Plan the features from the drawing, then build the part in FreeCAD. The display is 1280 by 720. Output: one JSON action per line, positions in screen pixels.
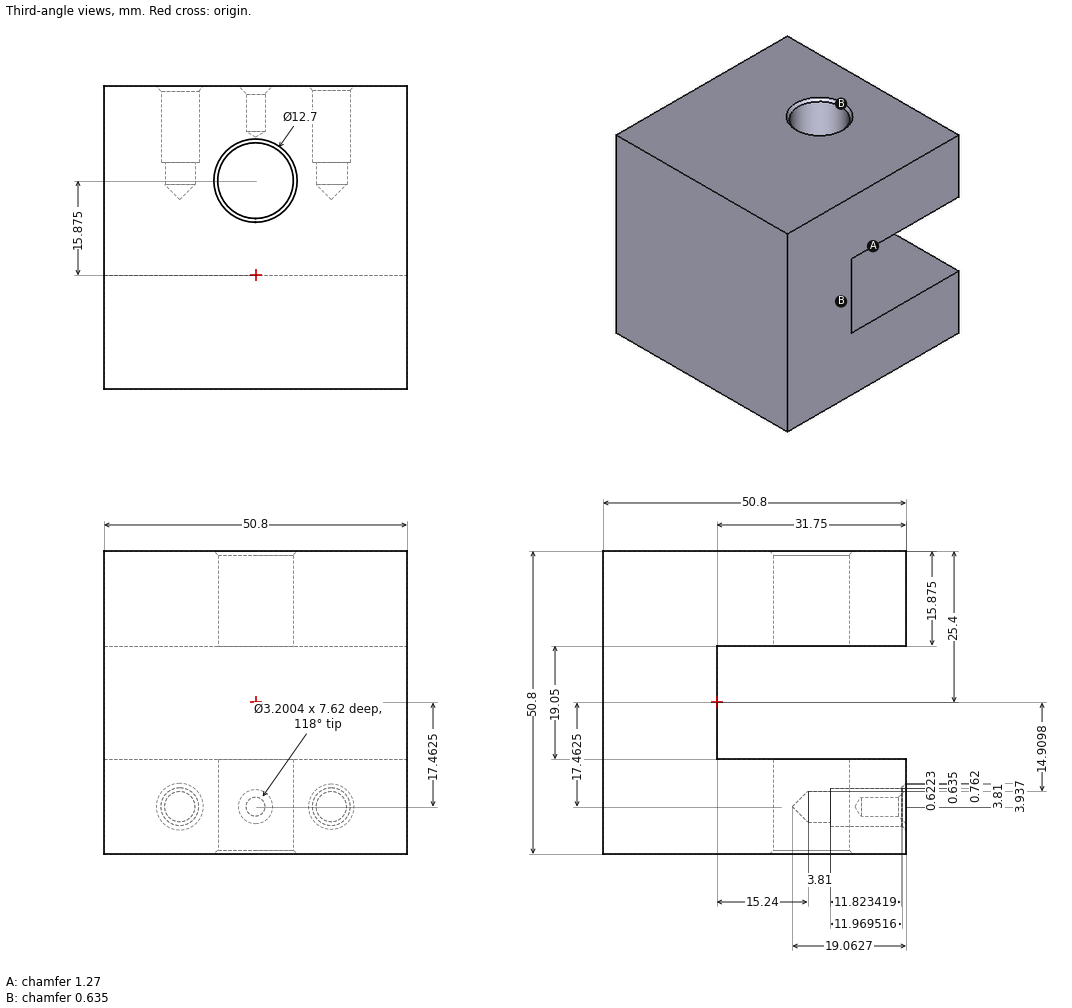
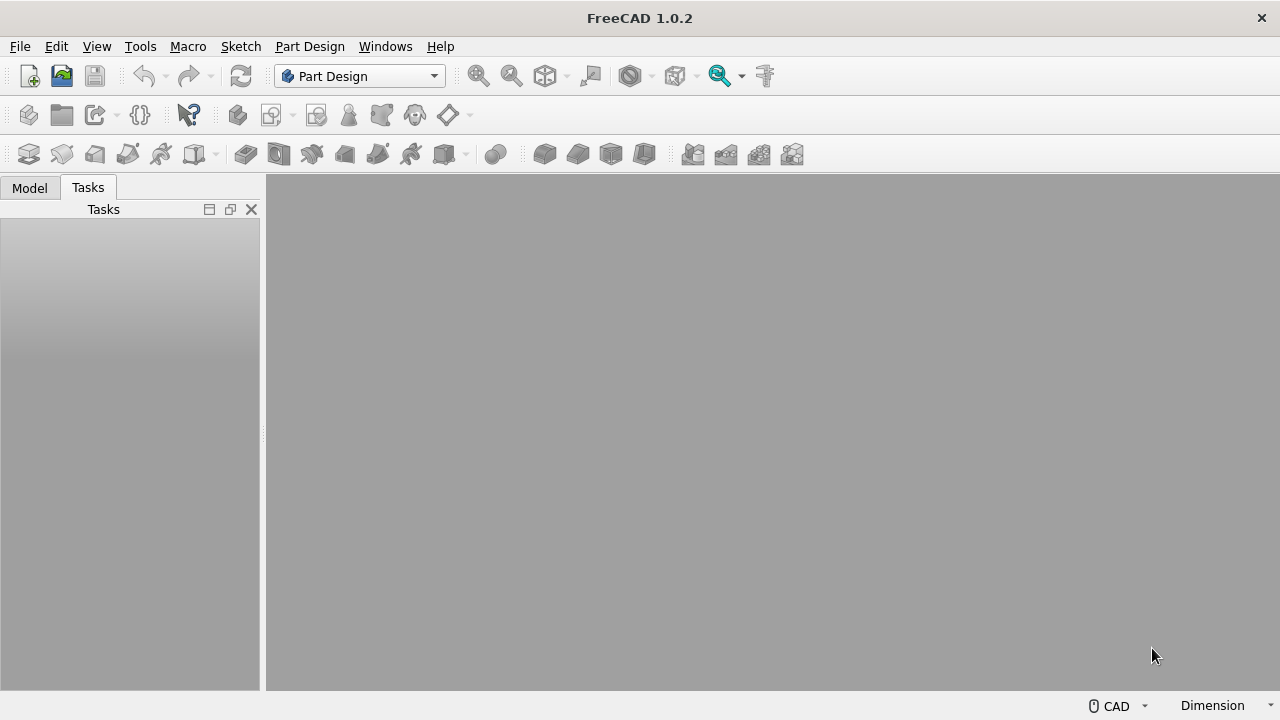
{"action": "left_click", "coordinate": [29, 76]}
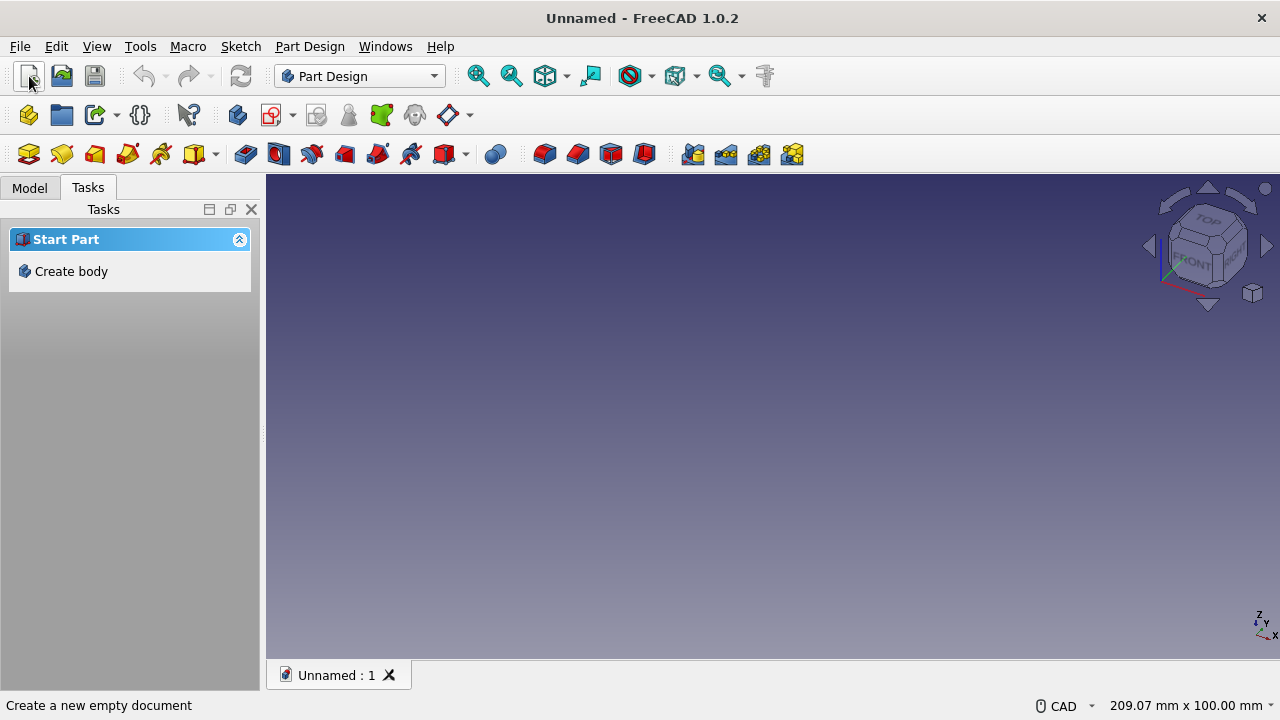
{"action": "left_click", "coordinate": [270, 116]}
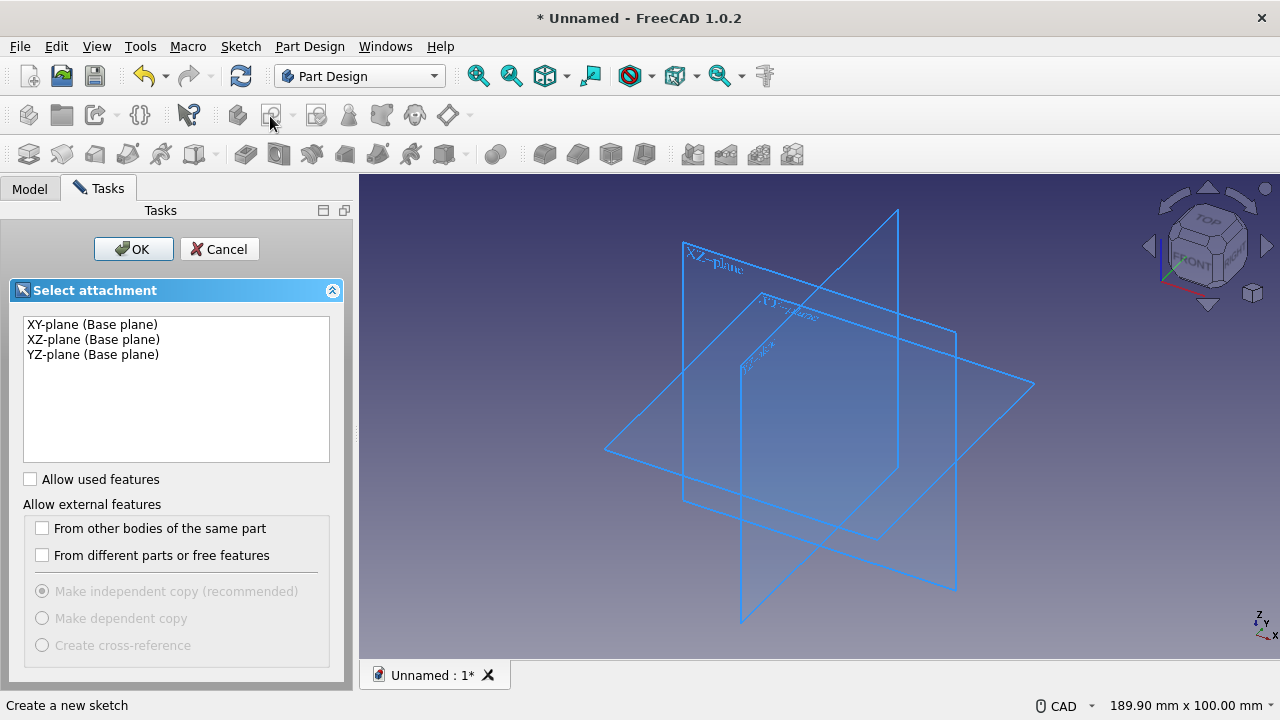
{"action": "left_click", "coordinate": [84, 354]}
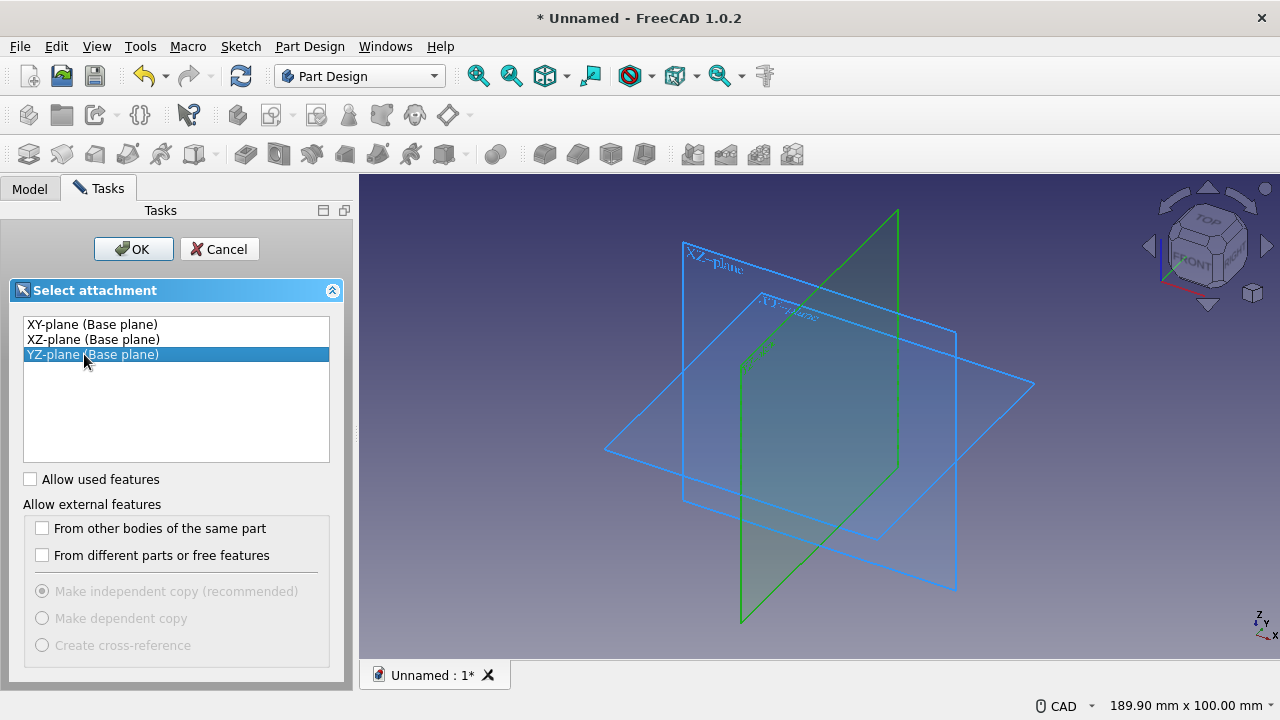
{"action": "left_click", "coordinate": [134, 249]}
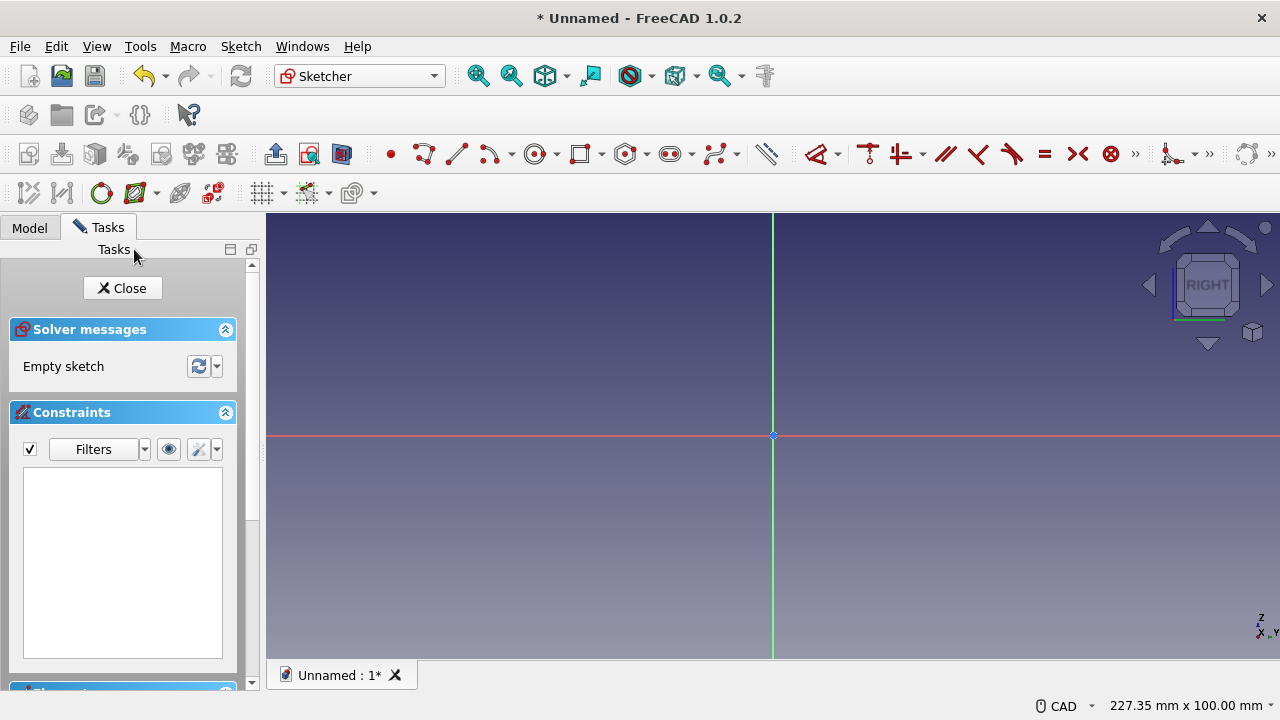
{"action": "left_click", "coordinate": [424, 154]}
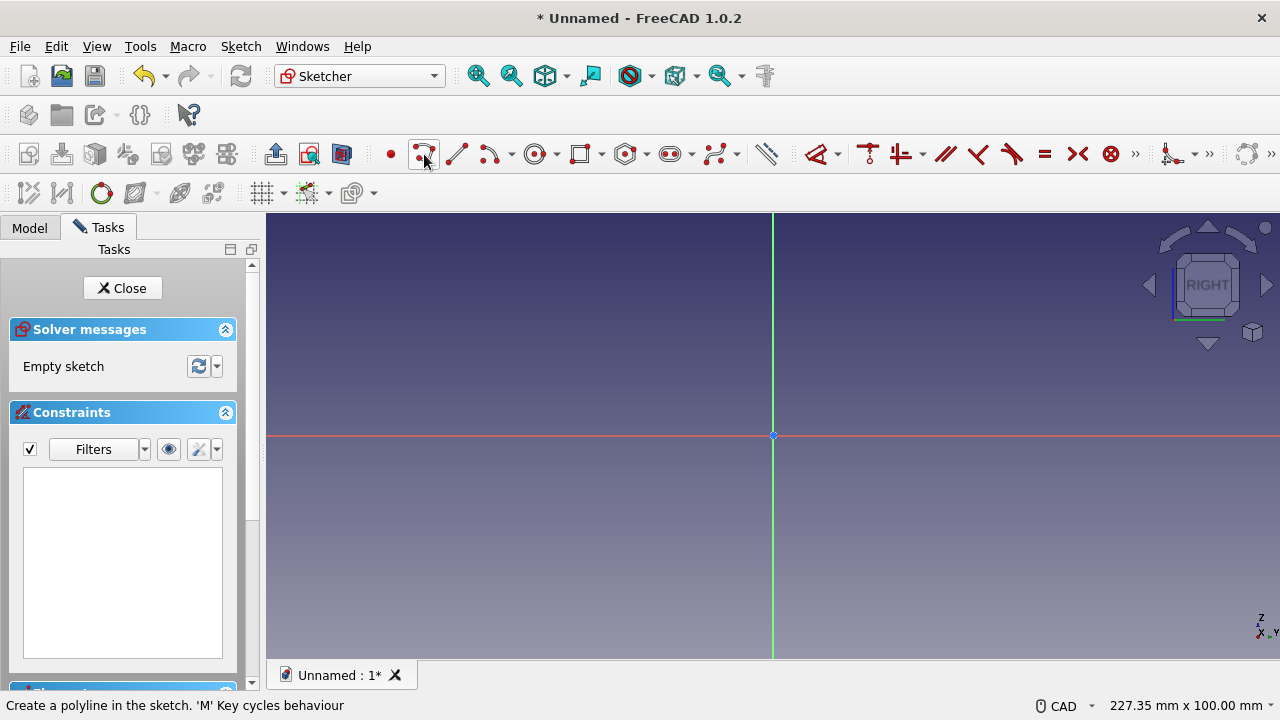
{"action": "left_click", "coordinate": [773, 478]}
{"action": "left_click", "coordinate": [782, 394]}
{"action": "left_click", "coordinate": [915, 394]}
{"action": "left_click", "coordinate": [915, 323]}
{"action": "left_click", "coordinate": [688, 323]}
{"action": "left_click", "coordinate": [688, 549]}
{"action": "left_click", "coordinate": [915, 549]}
{"action": "left_click", "coordinate": [915, 478]}
{"action": "left_click", "coordinate": [773, 479]}
{"action": "key", "text": "Escape"}
{"action": "key", "text": "Escape"}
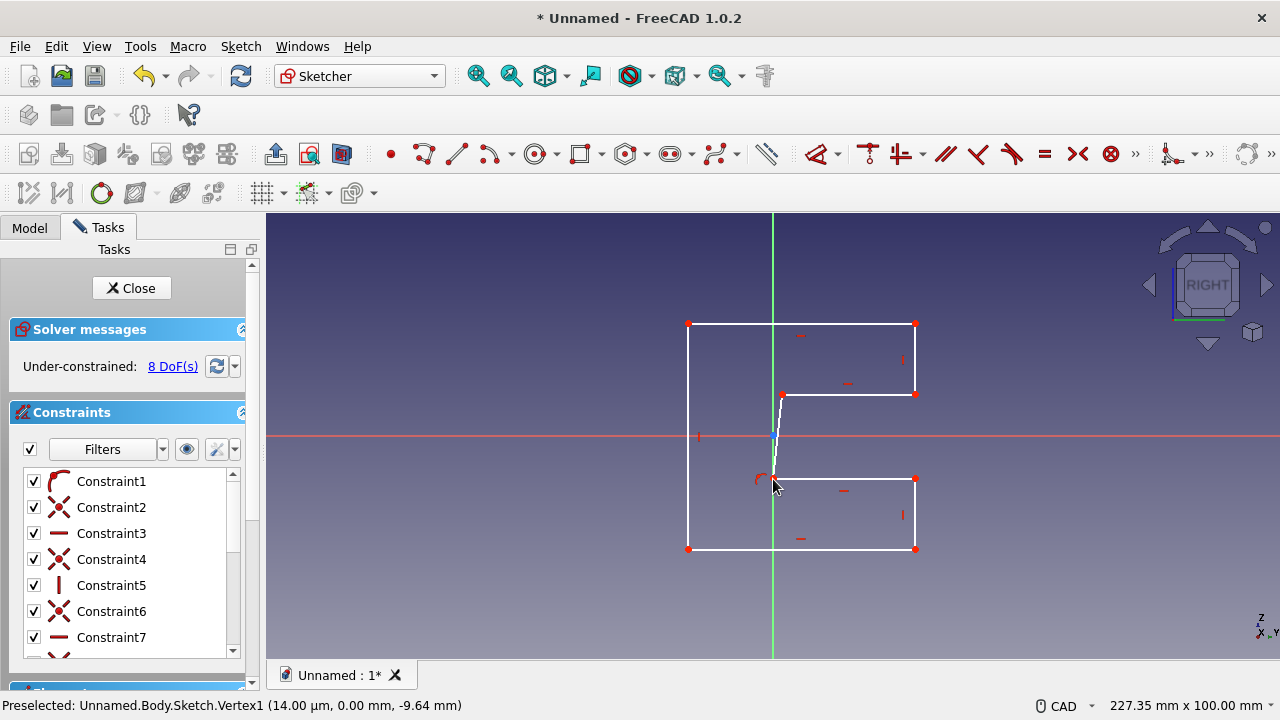
{"action": "left_click", "coordinate": [776, 454]}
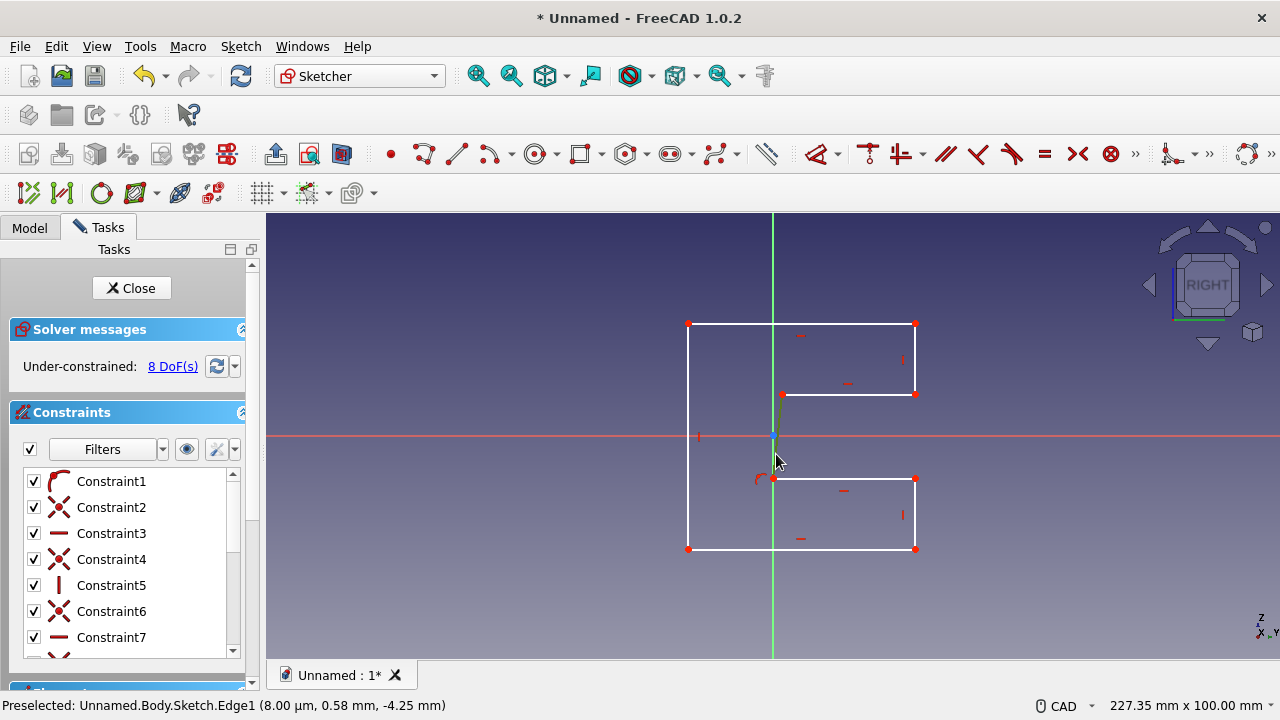
{"action": "key", "text": "v"}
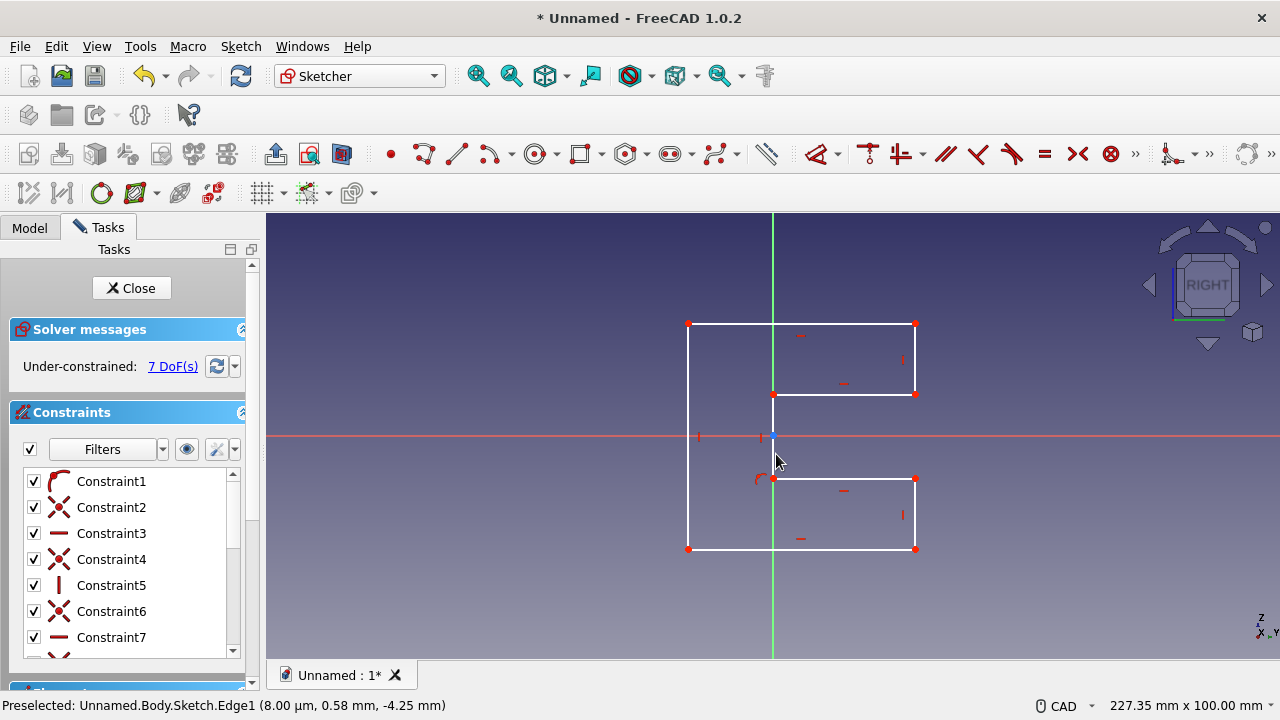
{"action": "left_click", "coordinate": [816, 154]}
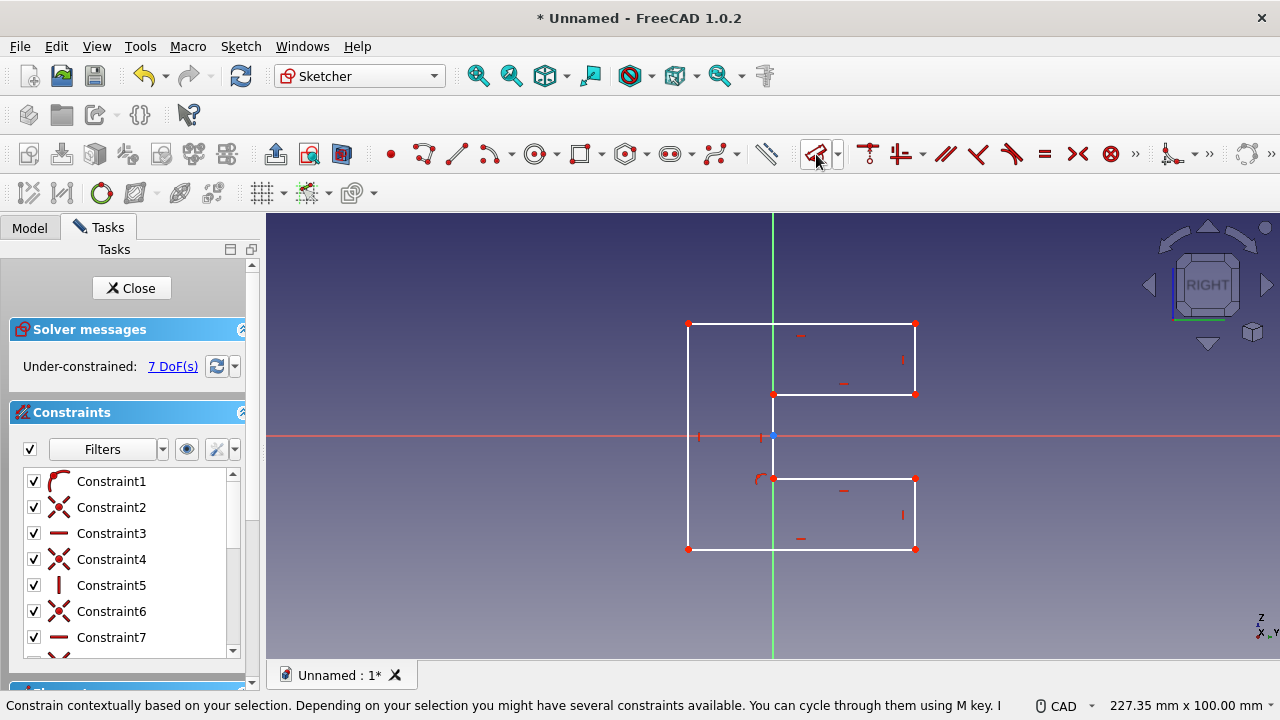
{"action": "left_click", "coordinate": [847, 324]}
{"action": "left_click", "coordinate": [802, 290]}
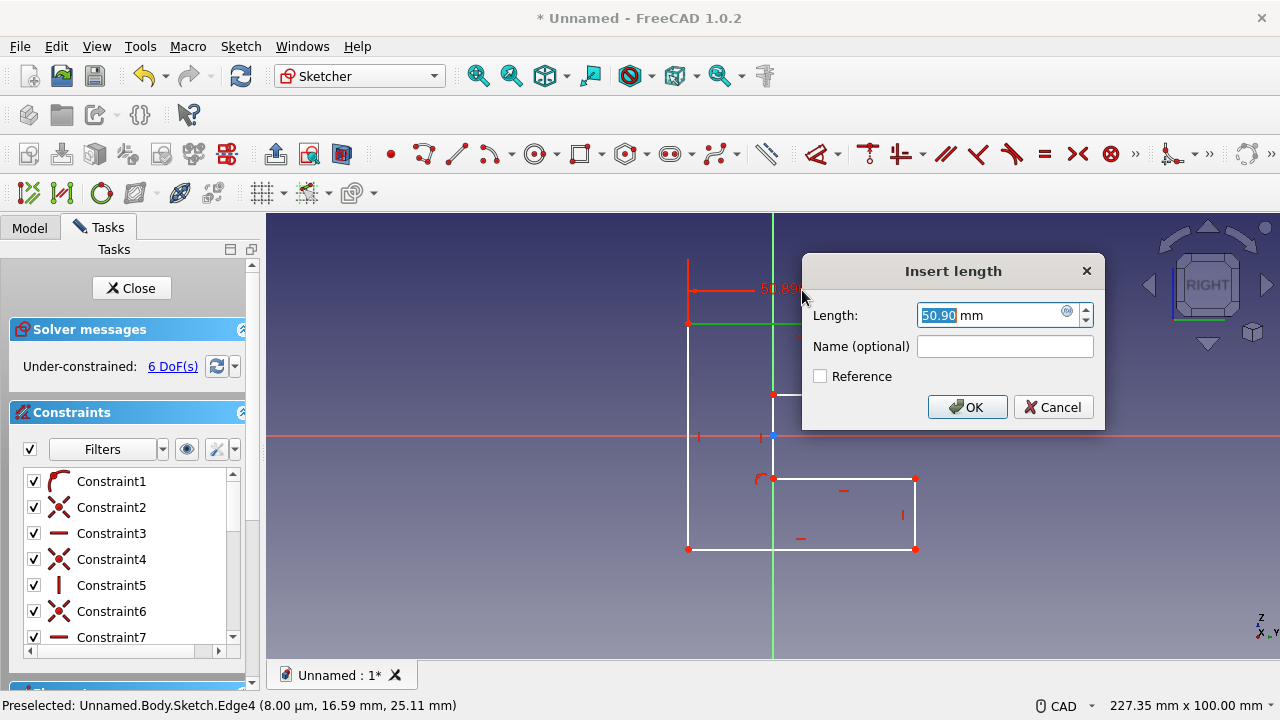
{"action": "type", "text": "50.8"}
{"action": "key", "text": "Return"}